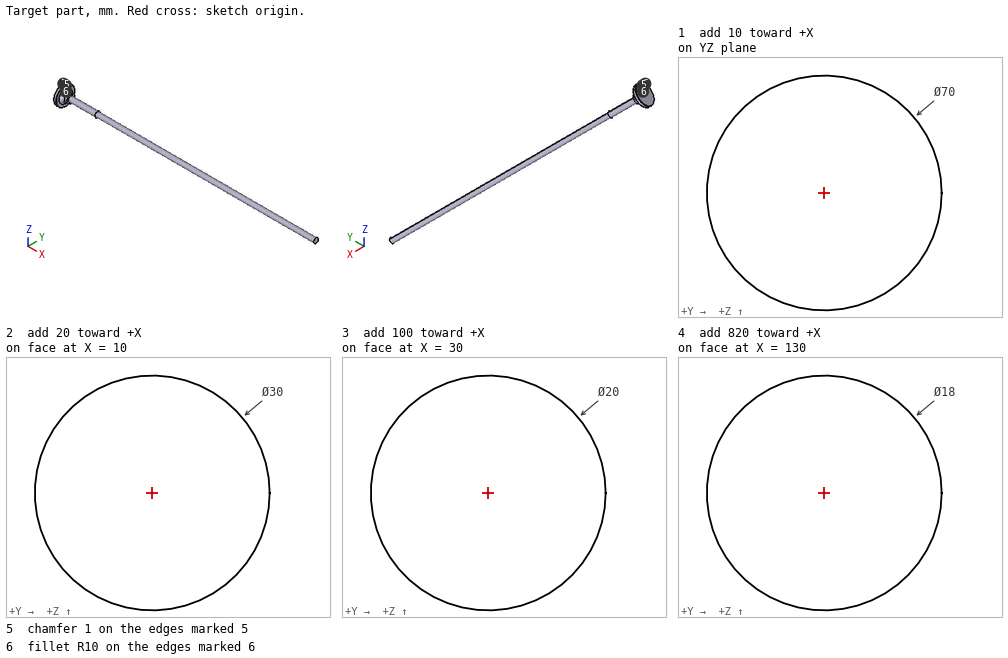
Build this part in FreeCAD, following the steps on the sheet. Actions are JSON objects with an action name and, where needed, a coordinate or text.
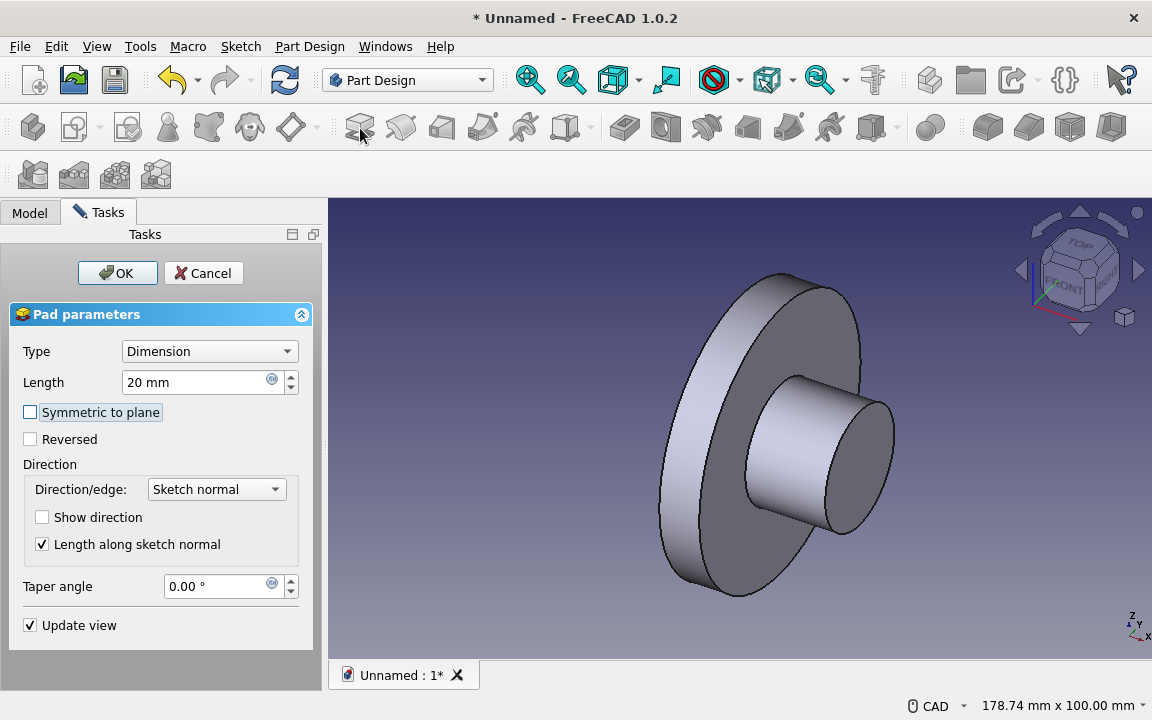
{"action": "left_click", "coordinate": [118, 273]}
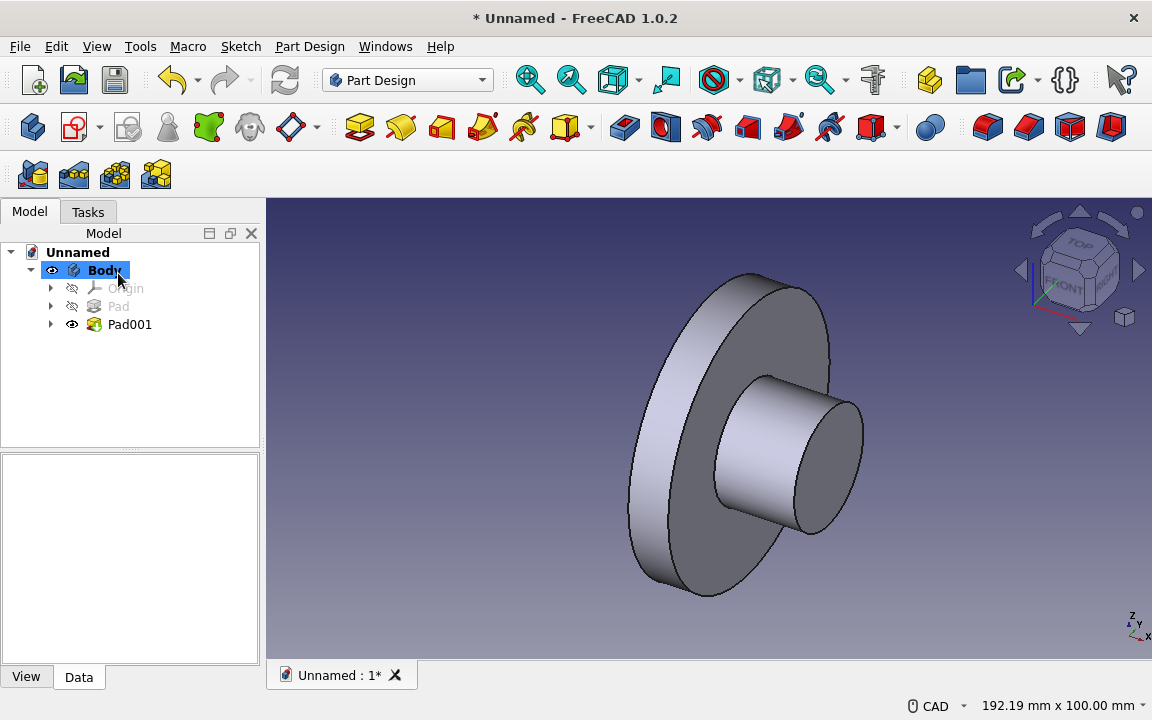
{"action": "left_click", "coordinate": [531, 80]}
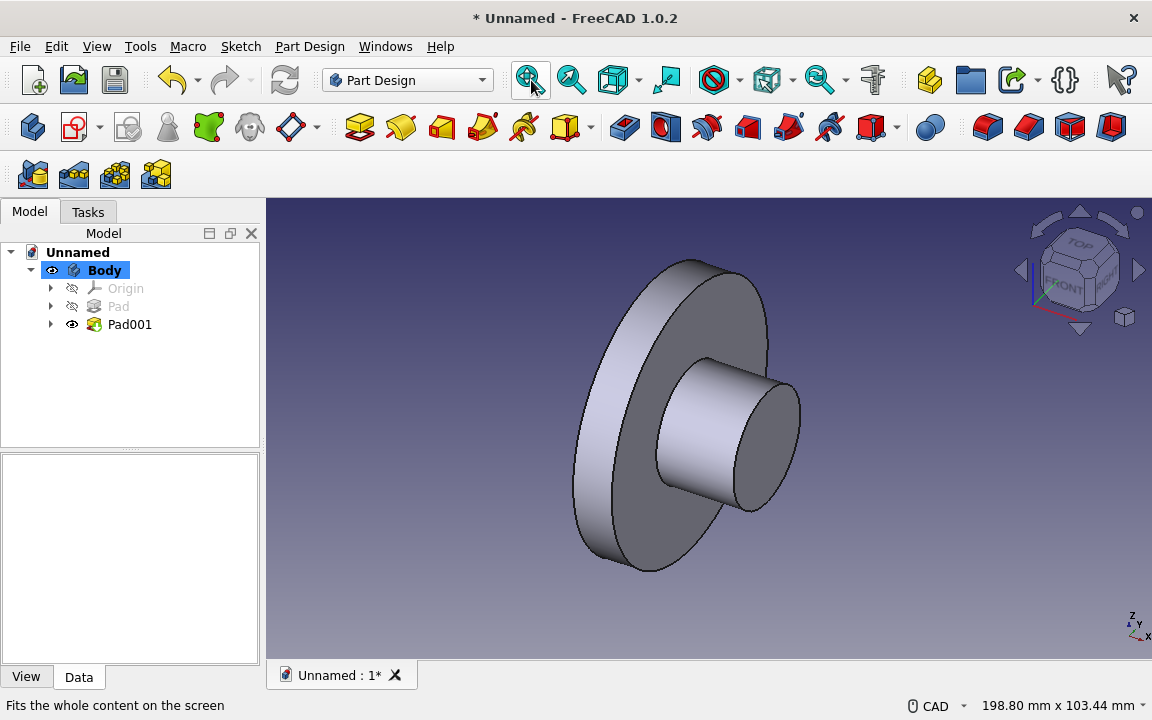
{"action": "left_click", "coordinate": [767, 447]}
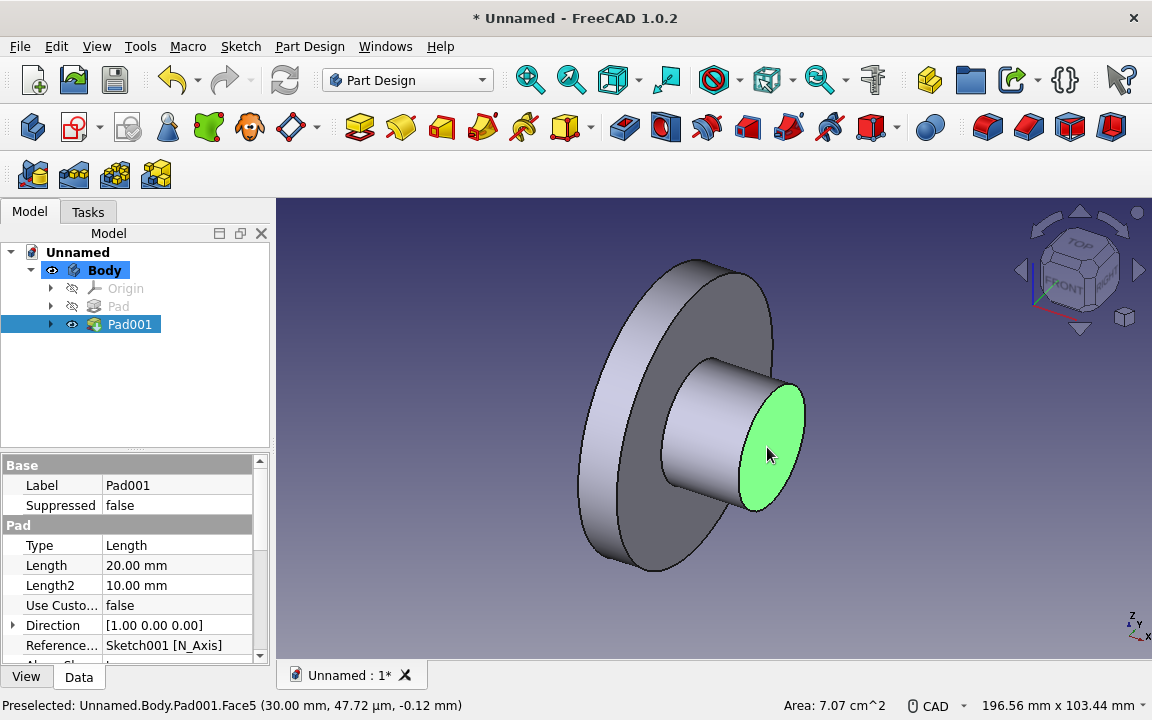
{"action": "left_click", "coordinate": [74, 128]}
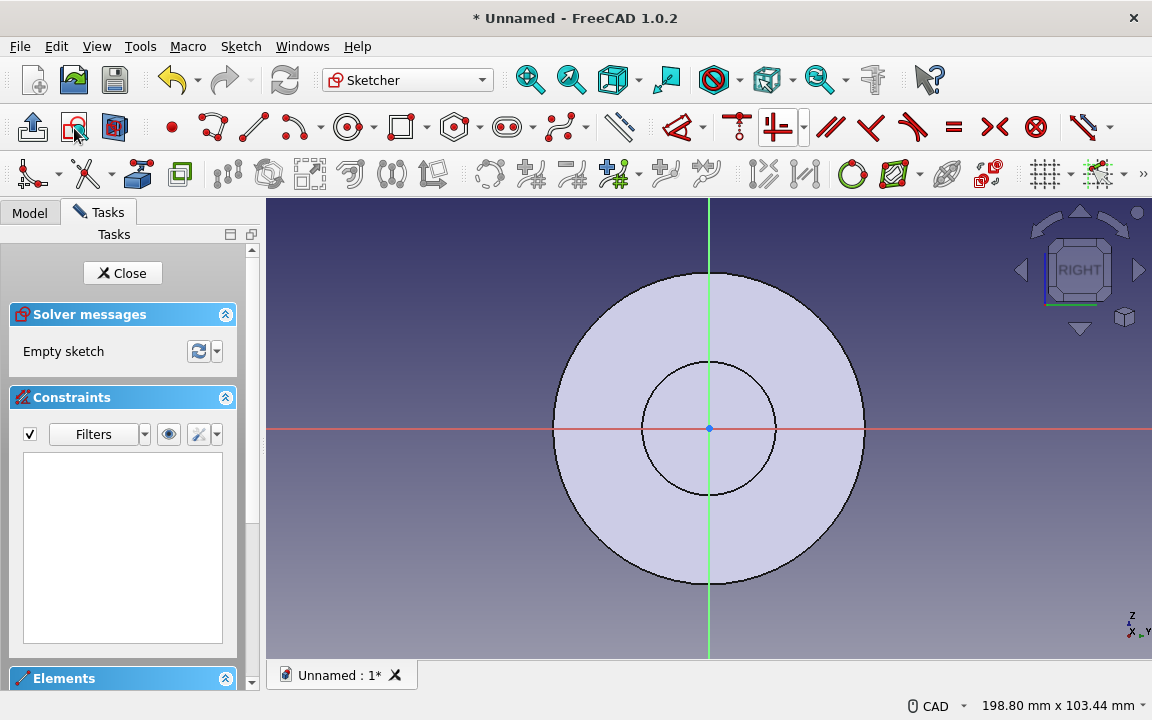
{"action": "scroll", "coordinate": [739, 428], "scroll_direction": "up", "scroll_amount": 6}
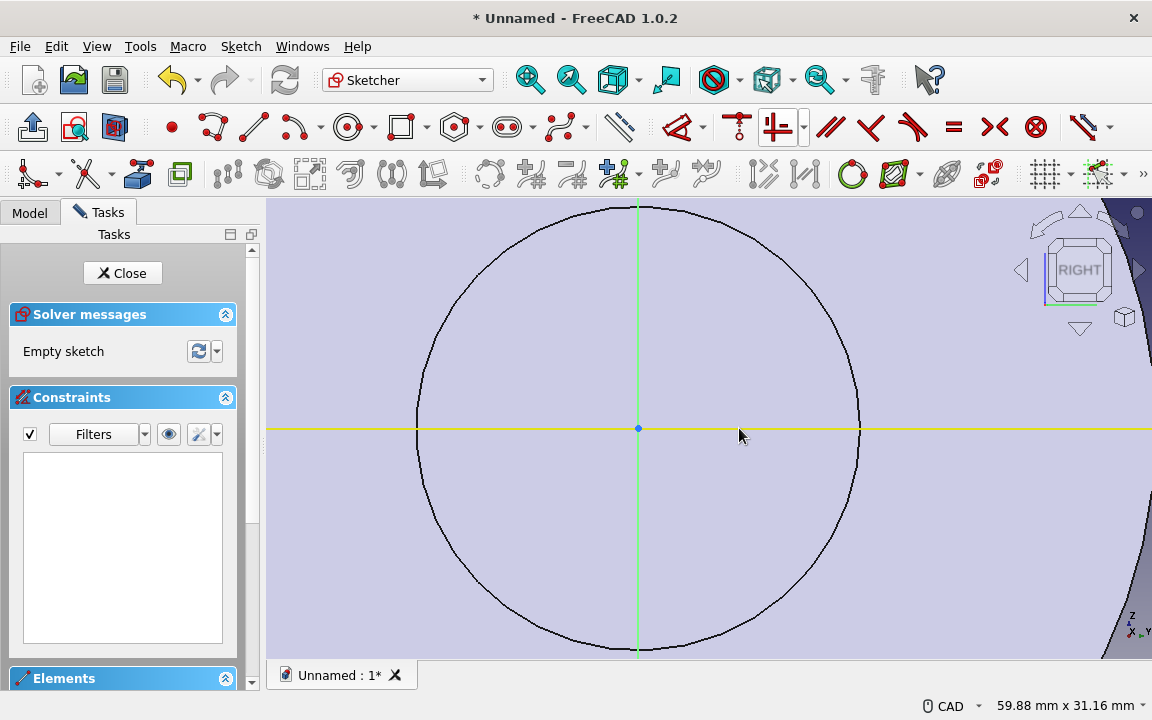
{"action": "left_click", "coordinate": [348, 128]}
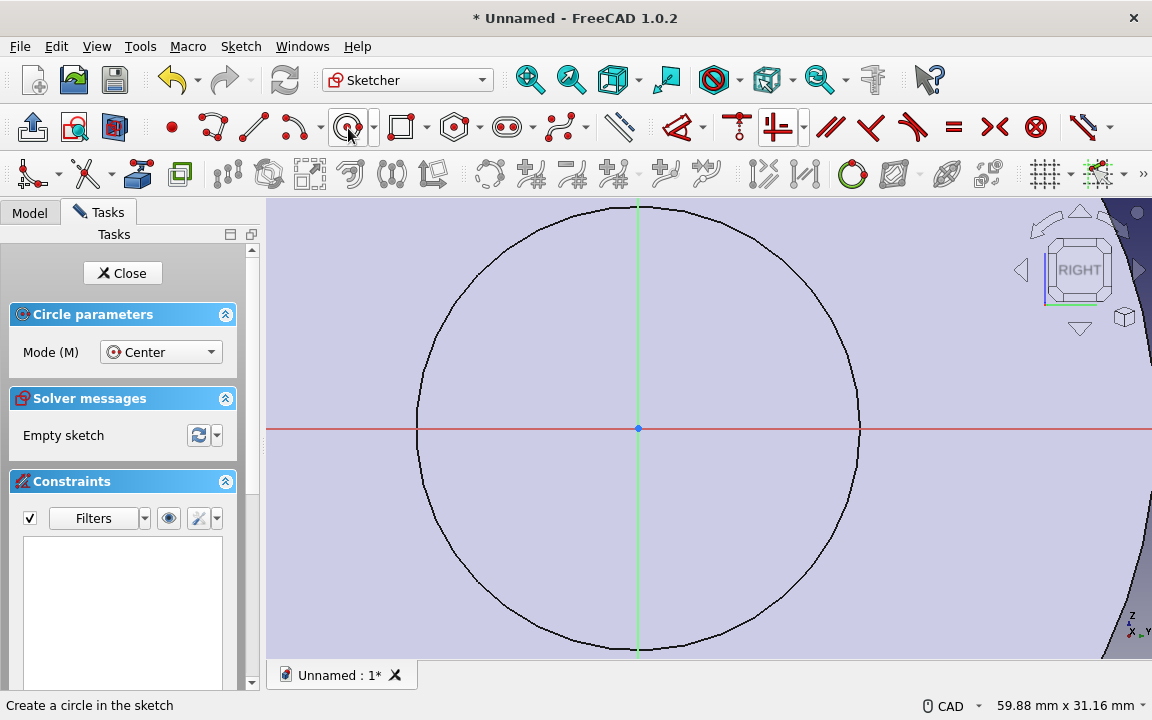
{"action": "left_click", "coordinate": [638, 428]}
{"action": "left_click", "coordinate": [743, 324]}
{"action": "key", "text": "Escape"}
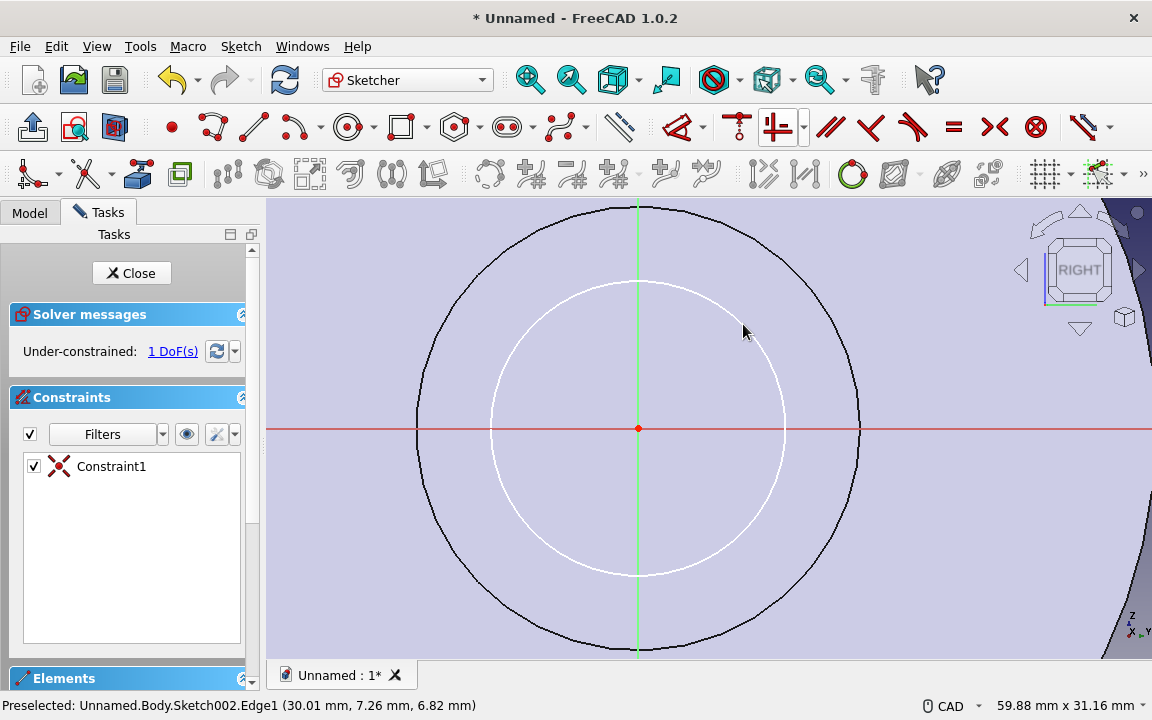
{"action": "key", "text": "d"}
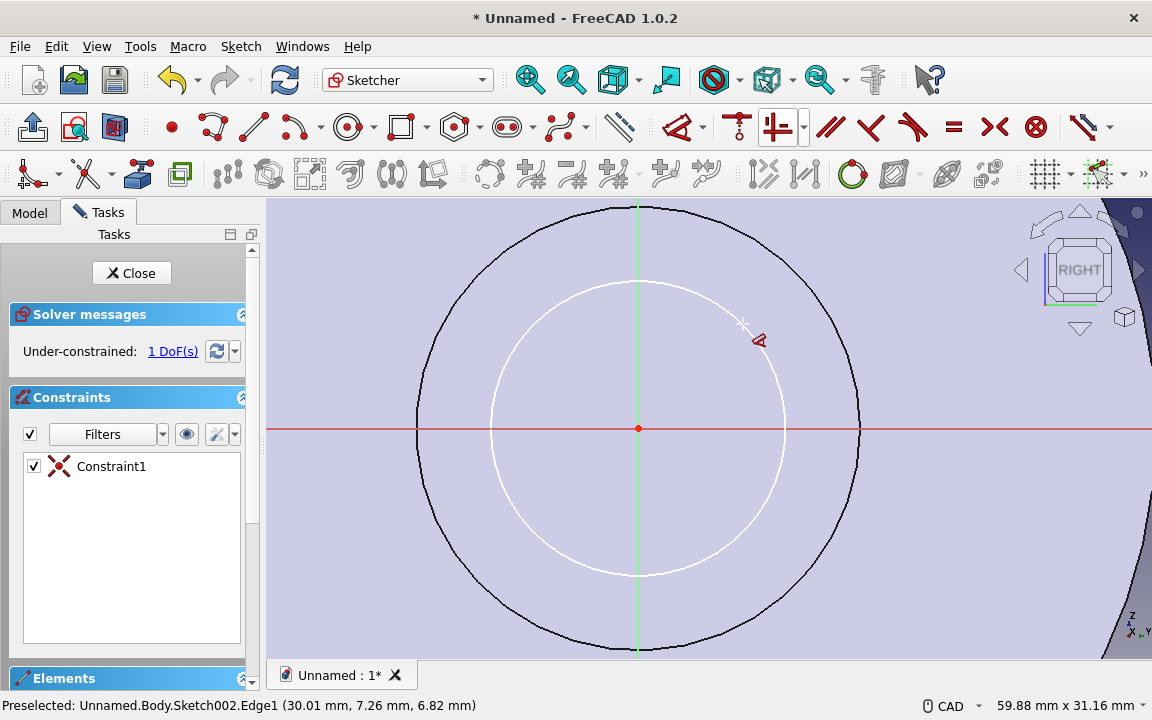
{"action": "left_click", "coordinate": [742, 324]}
{"action": "left_click", "coordinate": [765, 301]}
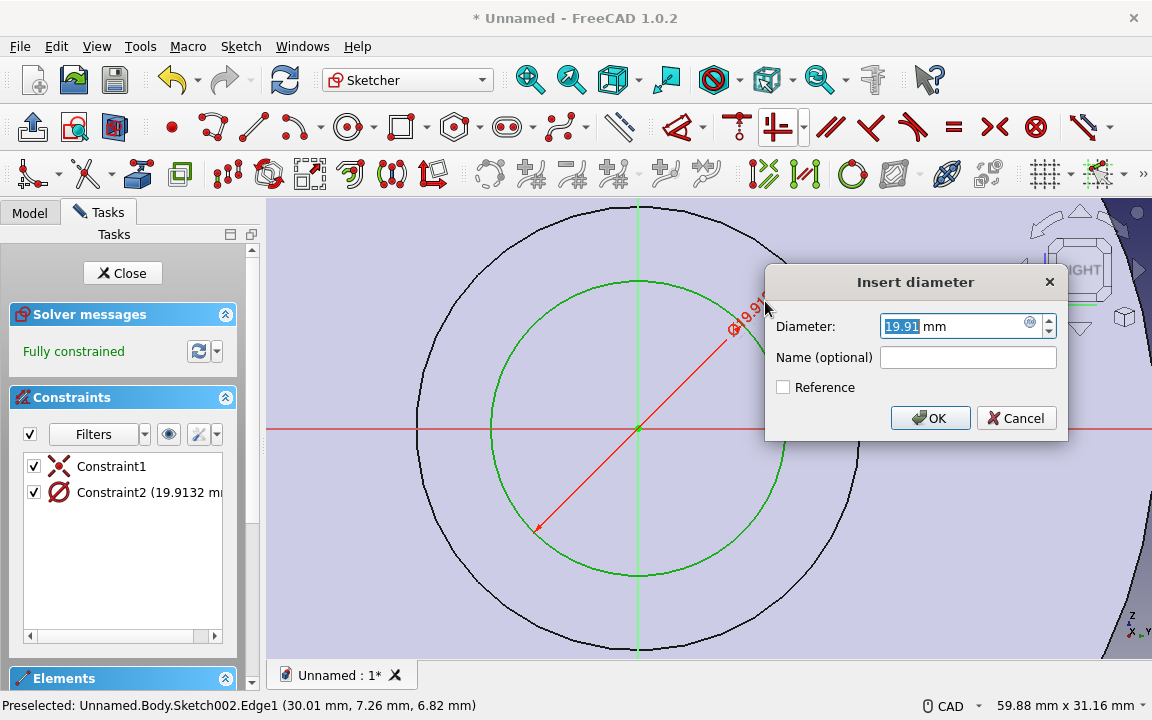
{"action": "type", "text": "20"}
{"action": "key", "text": "Return"}
{"action": "key", "text": "Escape"}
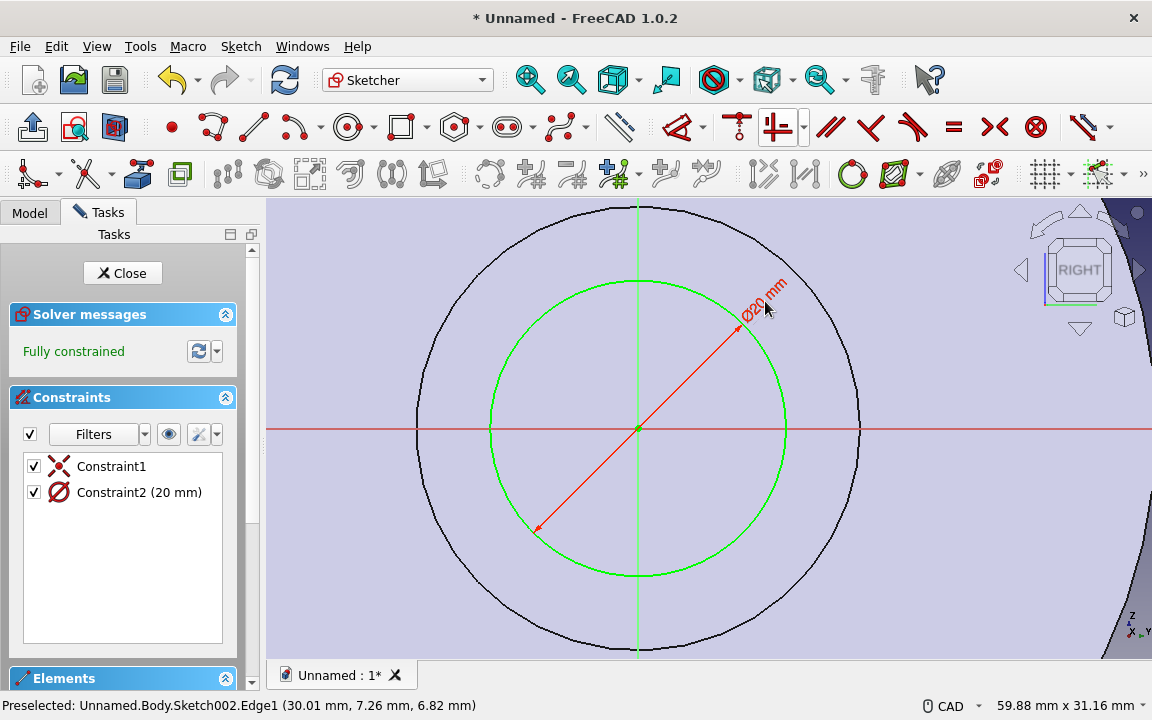
{"action": "left_click", "coordinate": [123, 273]}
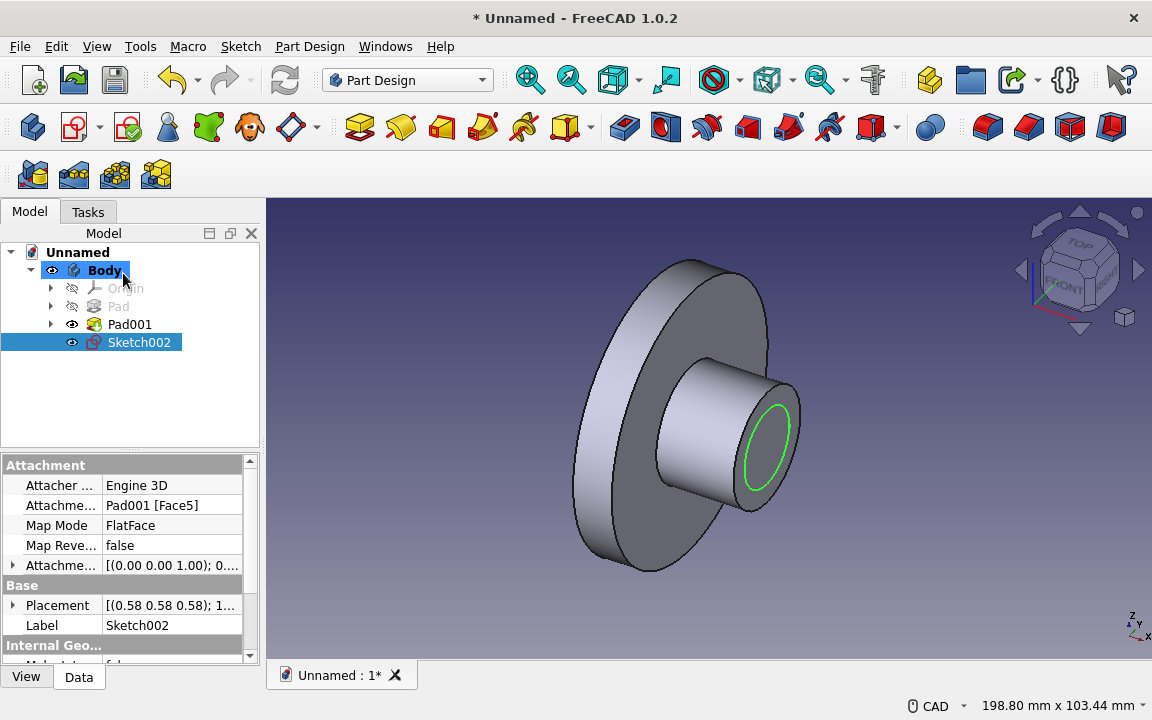
{"action": "left_click", "coordinate": [360, 128]}